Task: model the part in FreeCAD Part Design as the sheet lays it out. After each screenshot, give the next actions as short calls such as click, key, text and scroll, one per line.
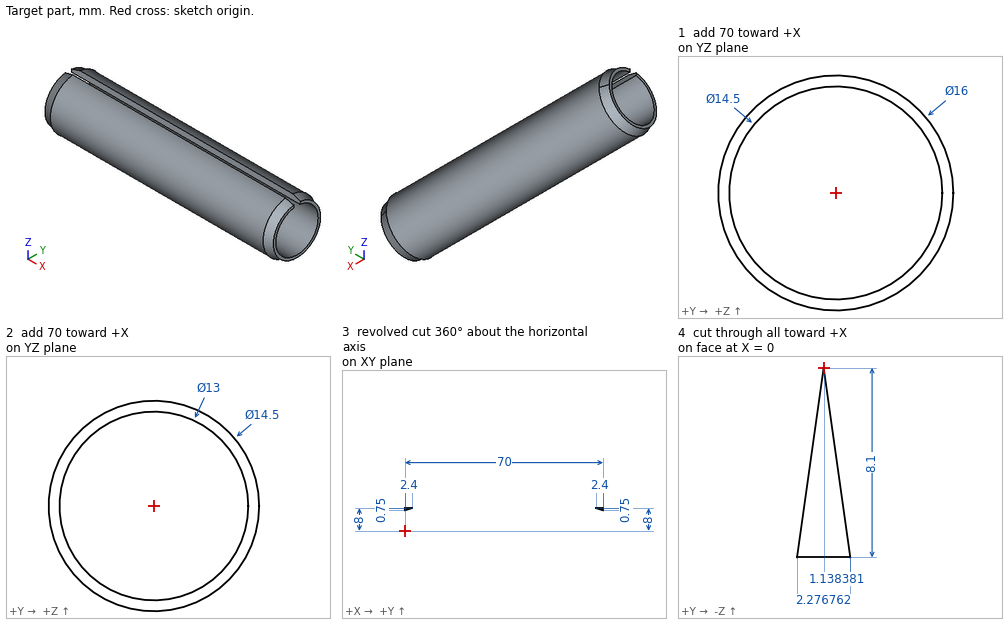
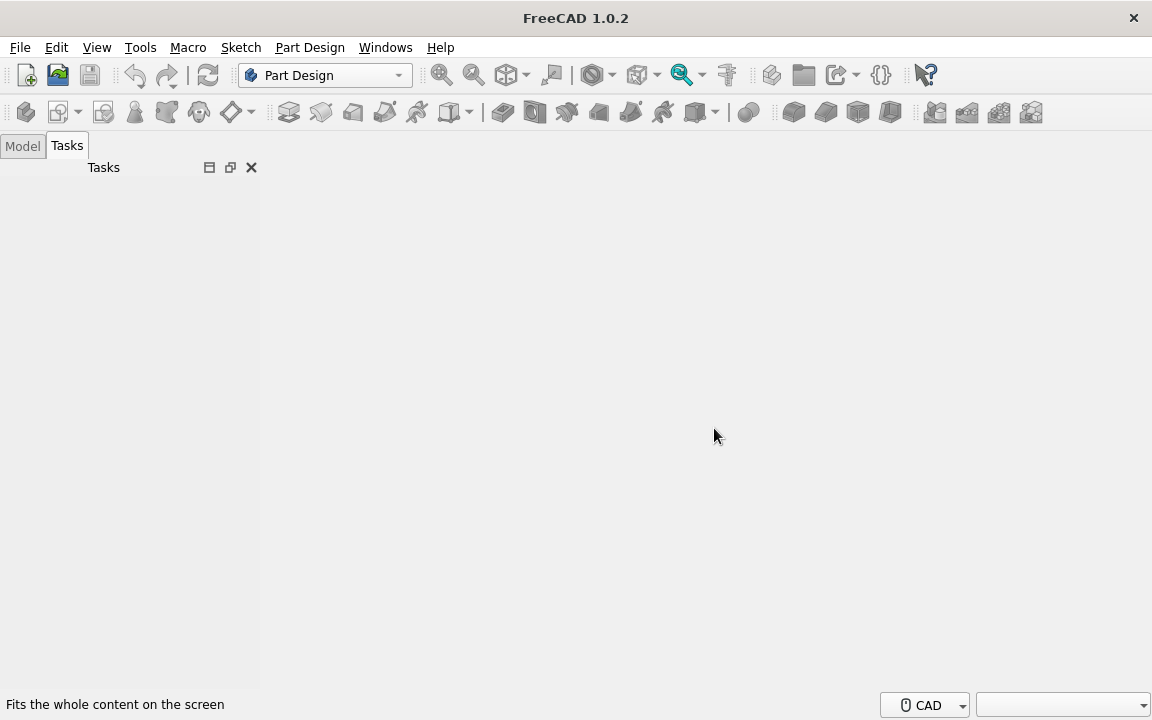
click(26, 76)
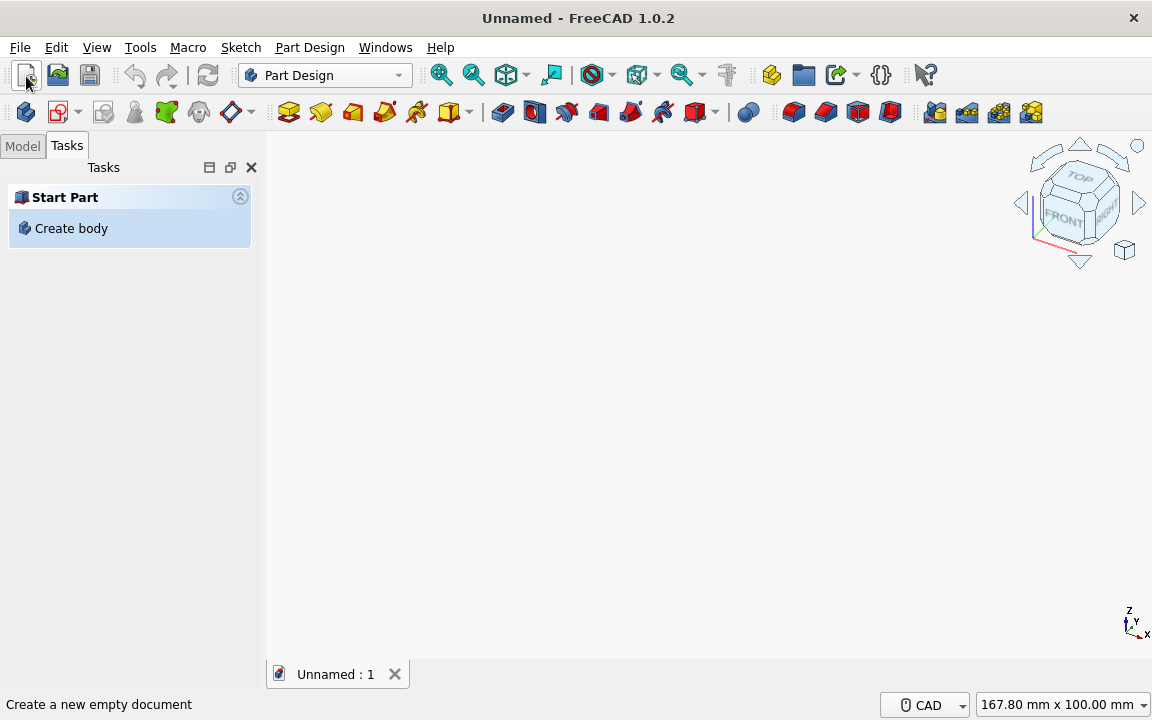
click(58, 112)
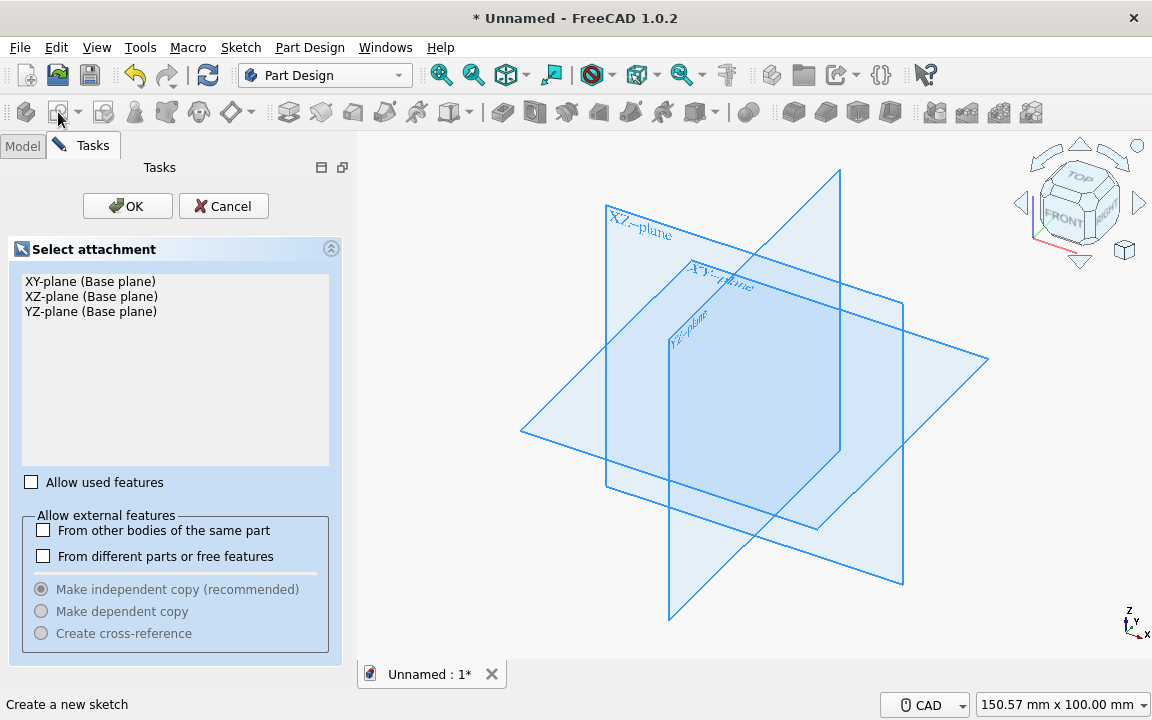
click(82, 312)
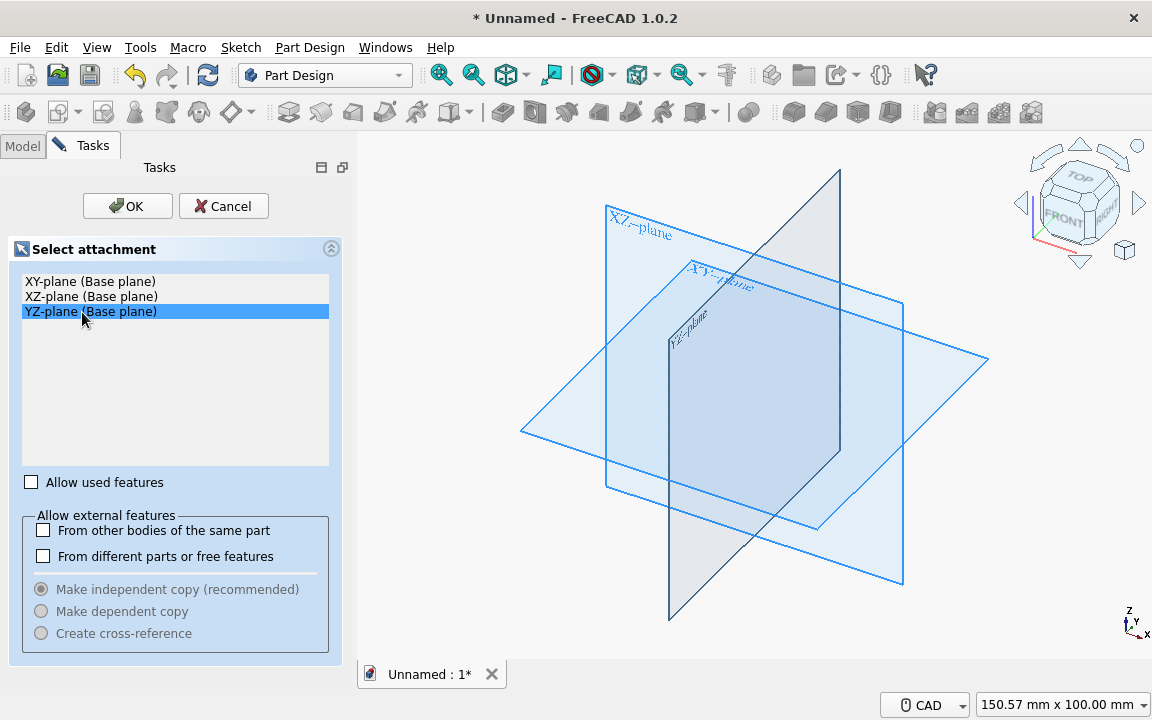
click(128, 206)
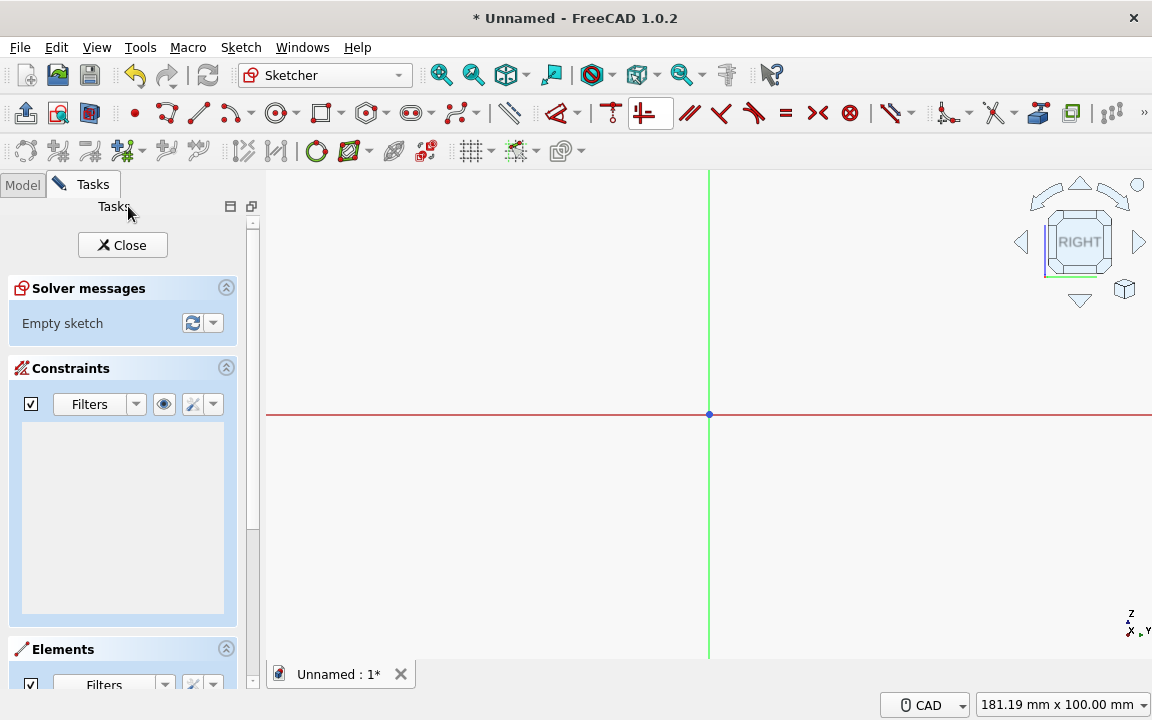
scroll(731, 415, up, 7)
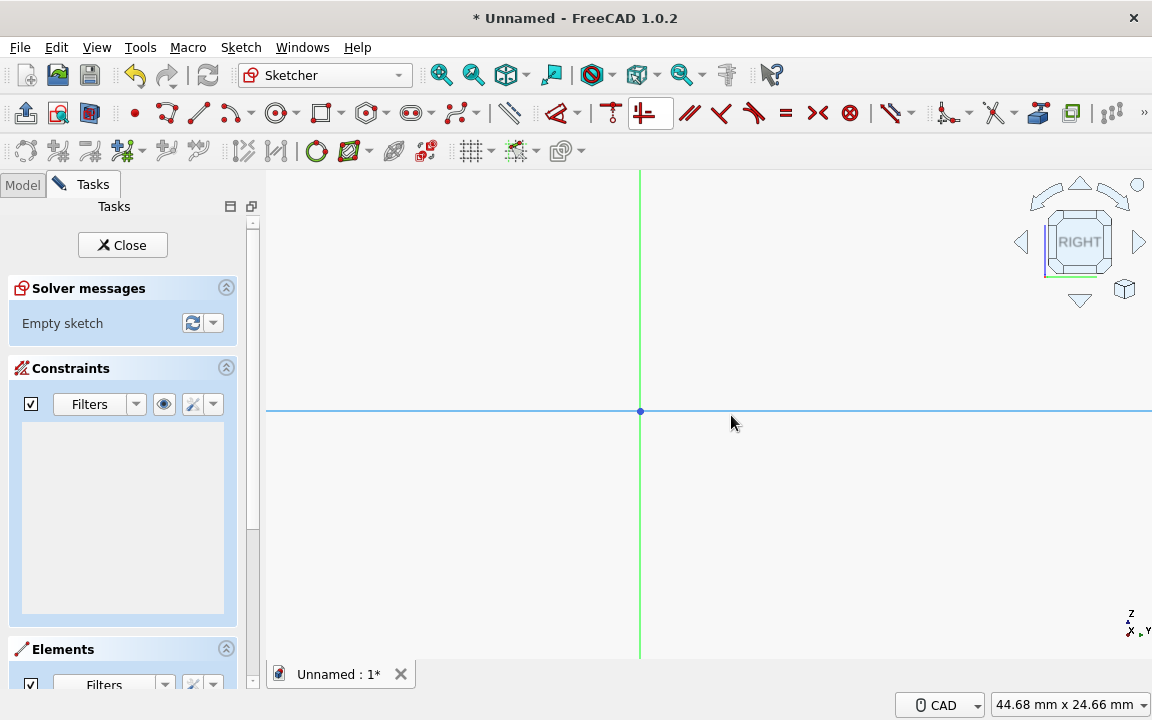
click(276, 114)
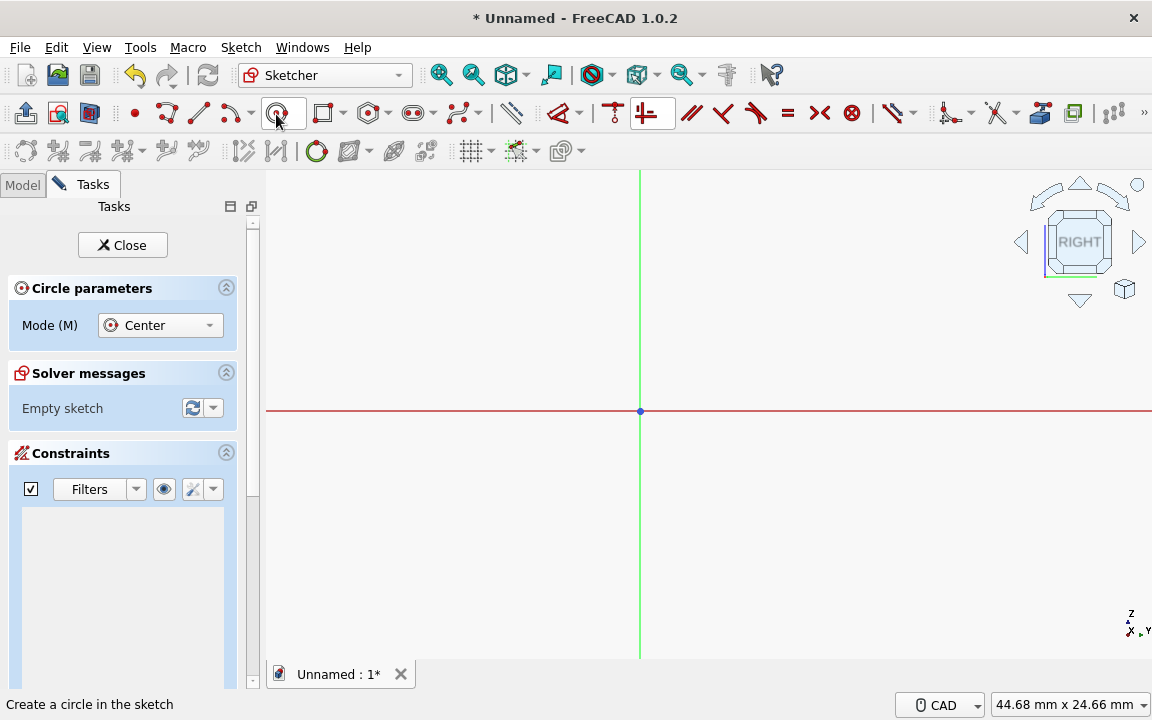
click(640, 411)
click(752, 299)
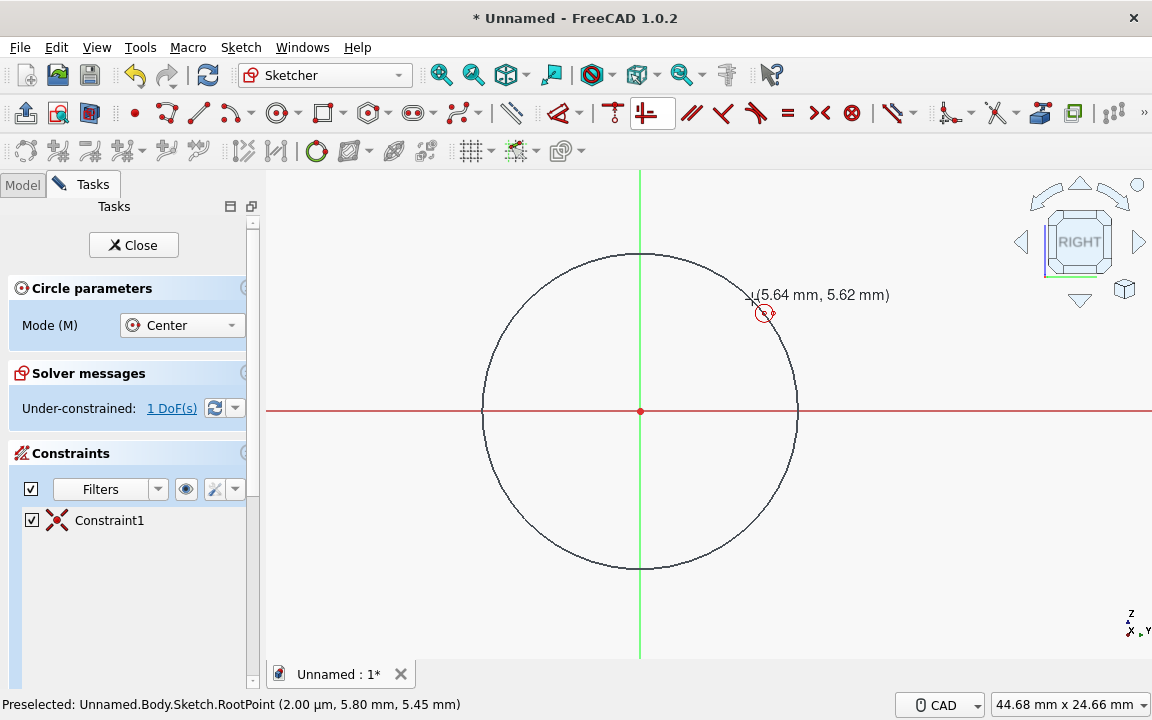
click(640, 411)
click(742, 310)
key(Escape)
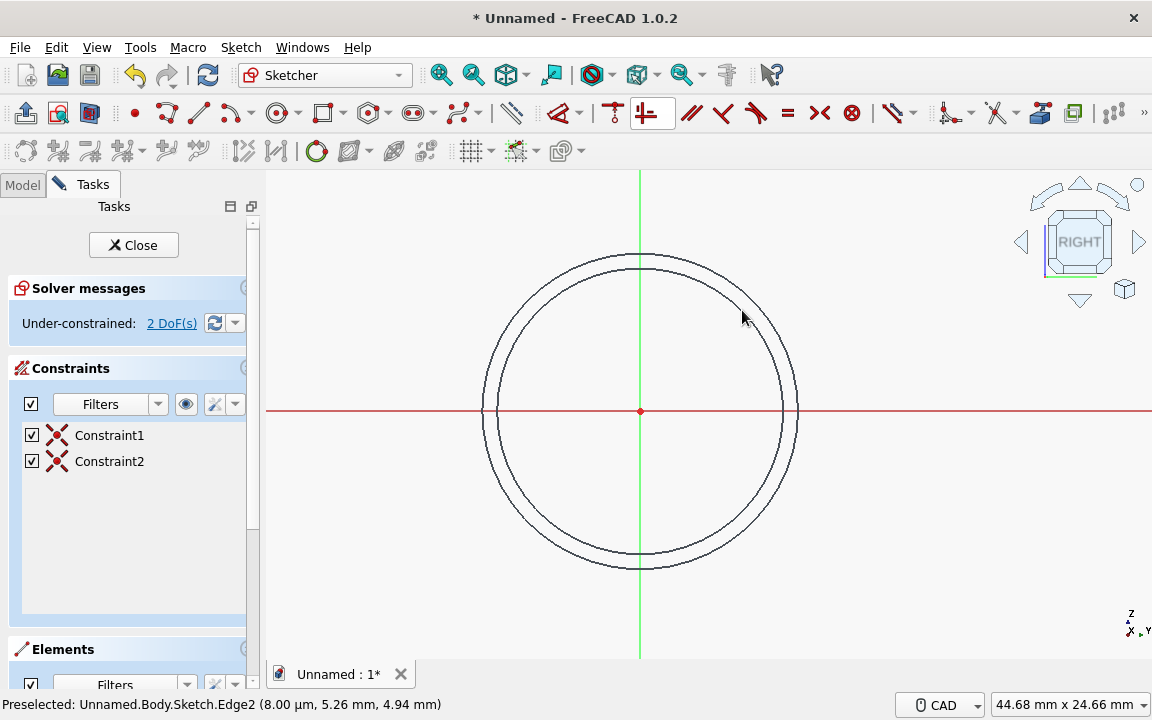
click(558, 114)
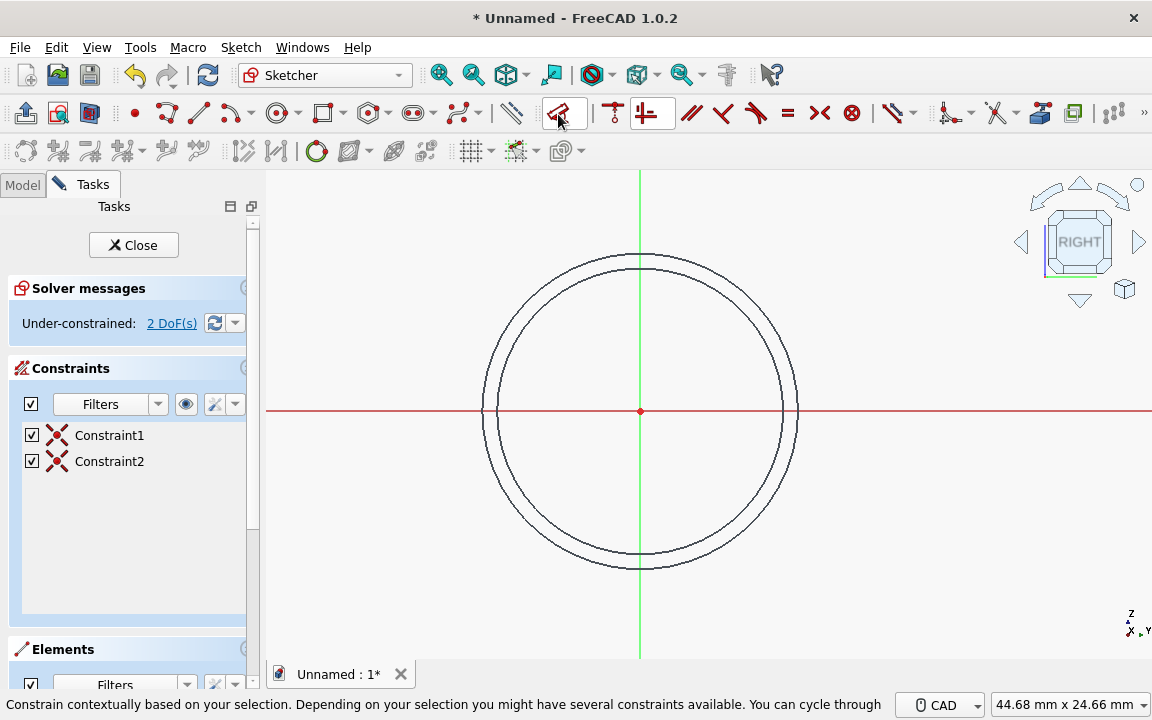
click(751, 299)
click(773, 276)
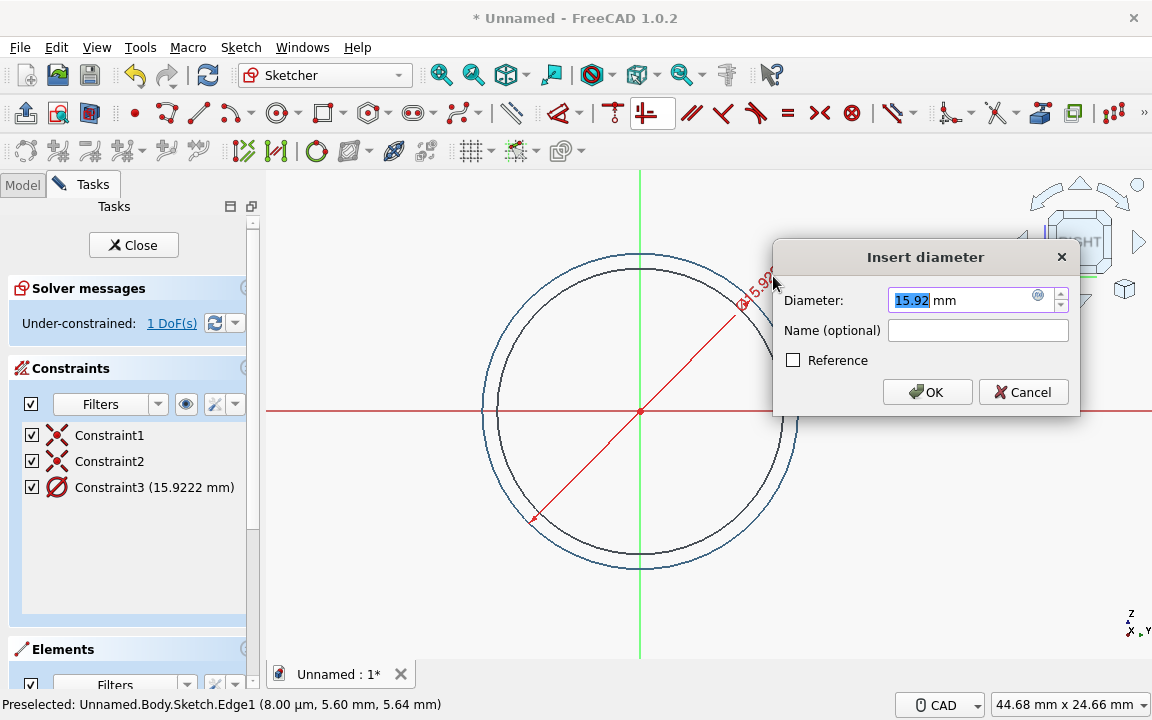
text(16)
key(Return)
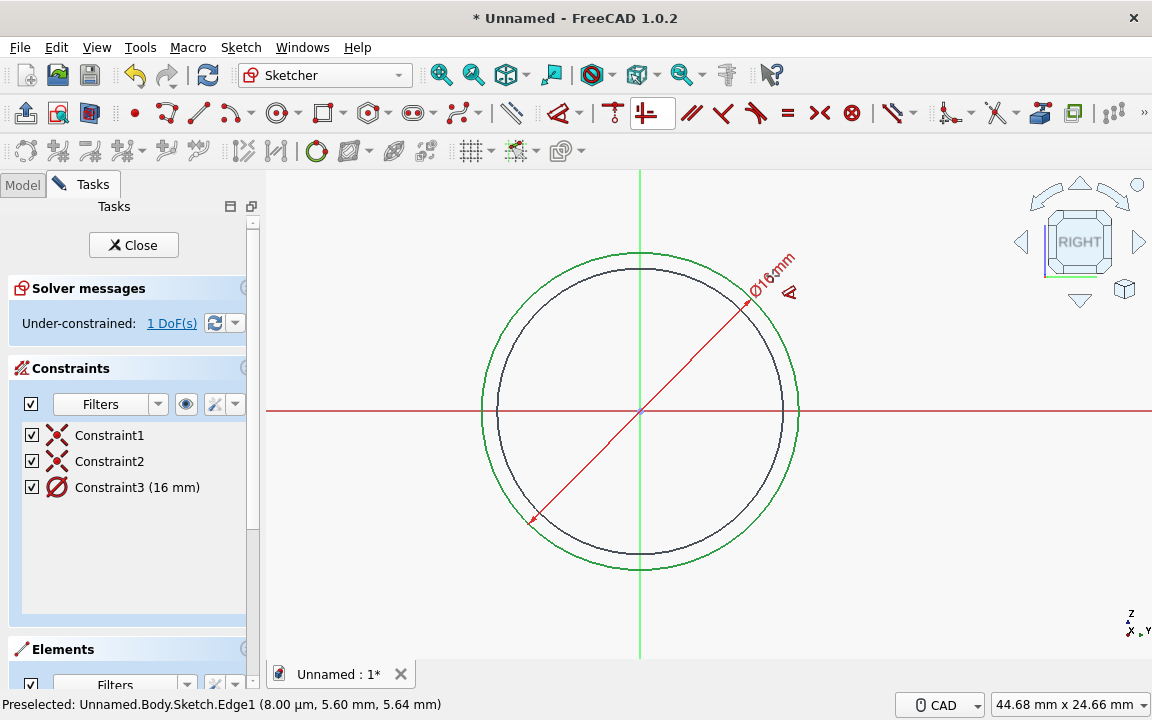
click(741, 310)
click(808, 362)